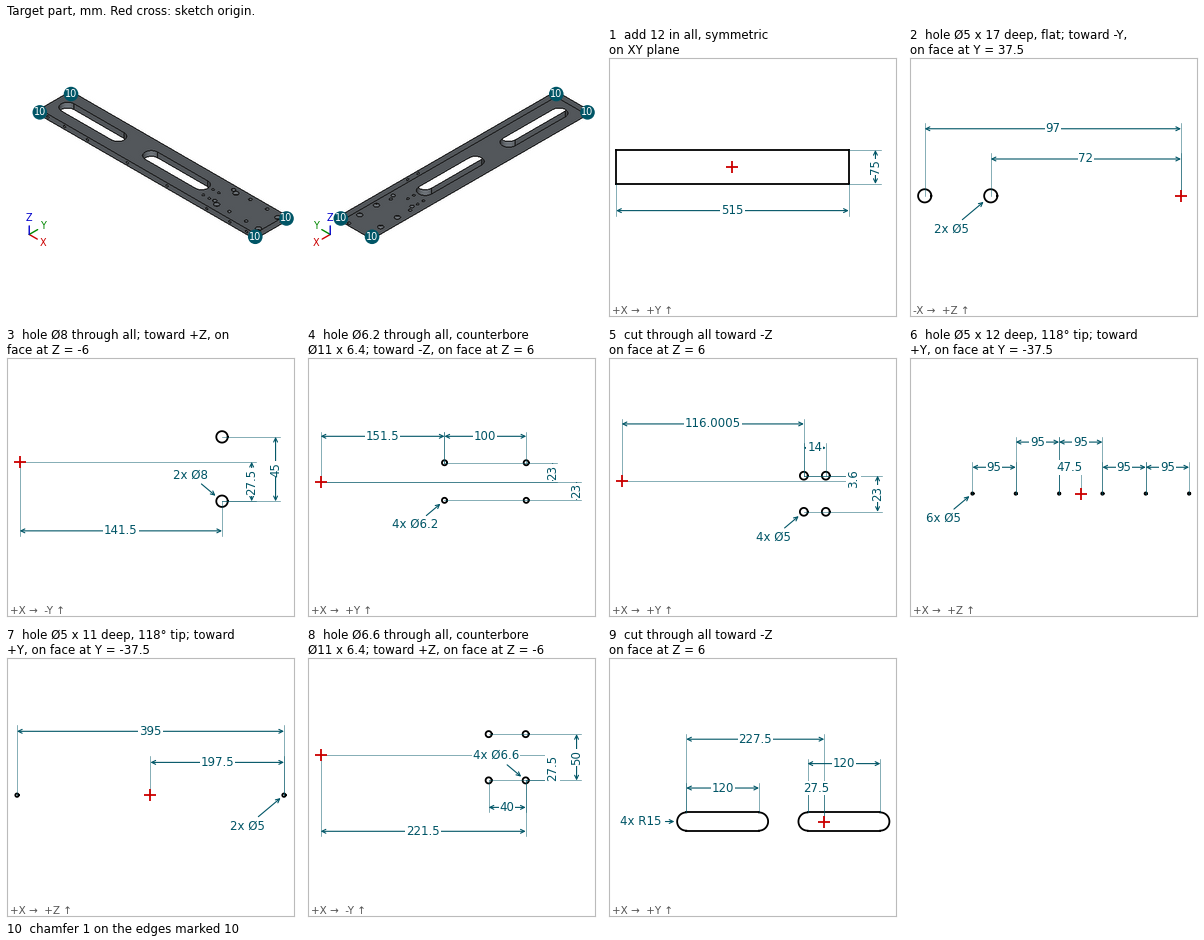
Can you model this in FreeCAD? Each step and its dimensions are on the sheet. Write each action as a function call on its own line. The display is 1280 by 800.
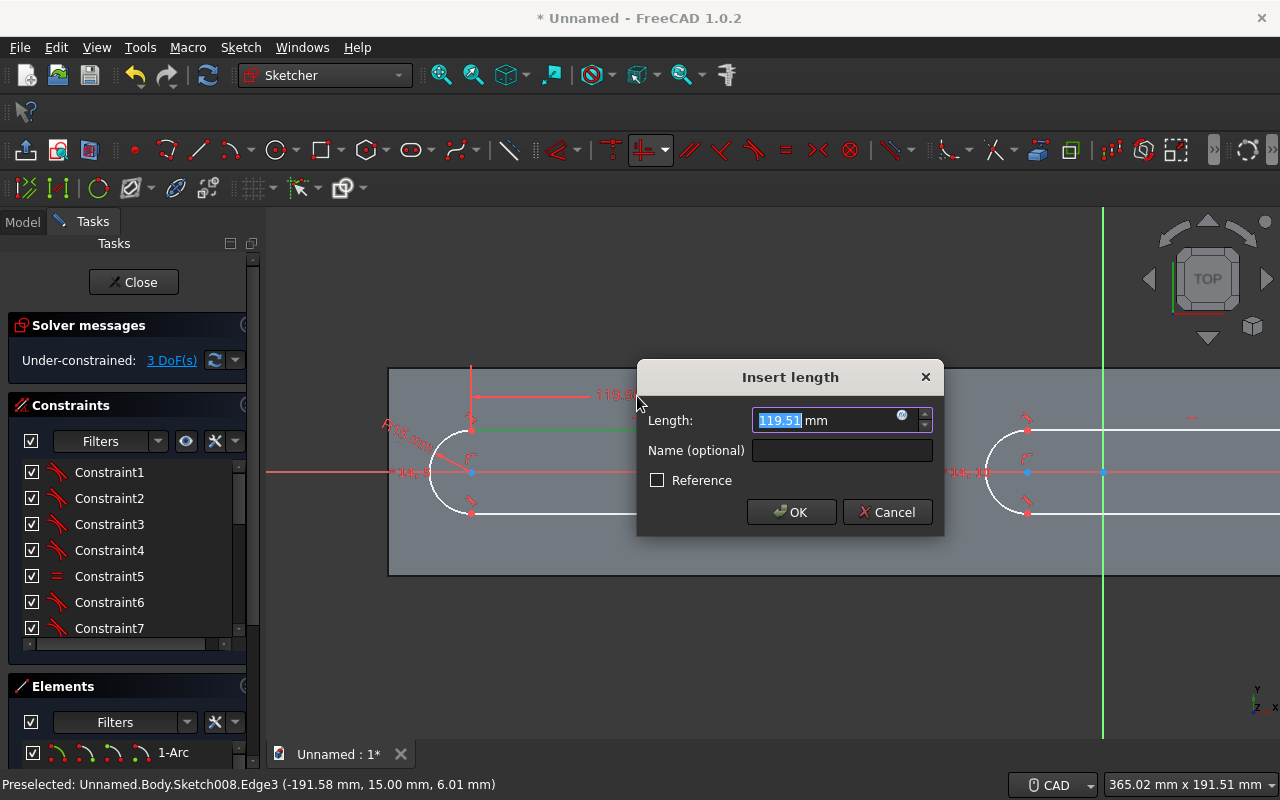
text(120)
key(Return)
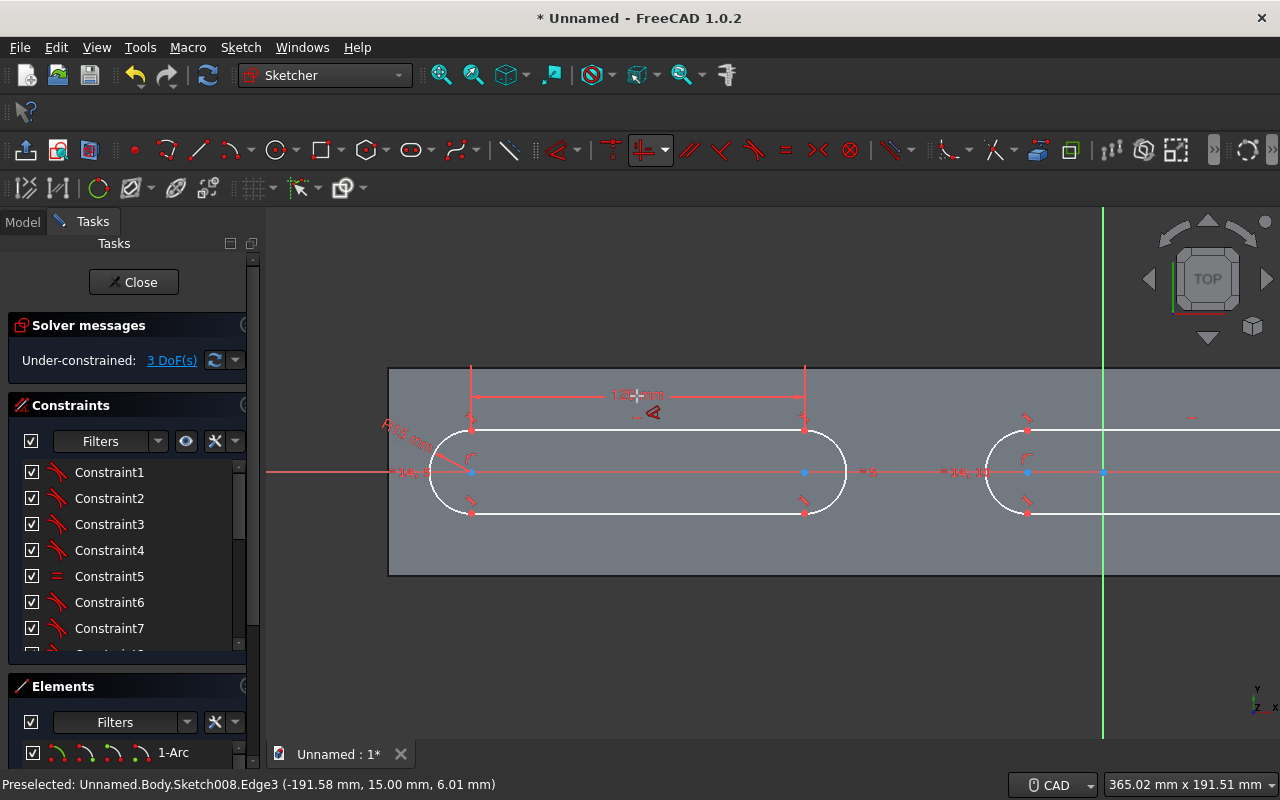
scroll(1094, 430, up, 2)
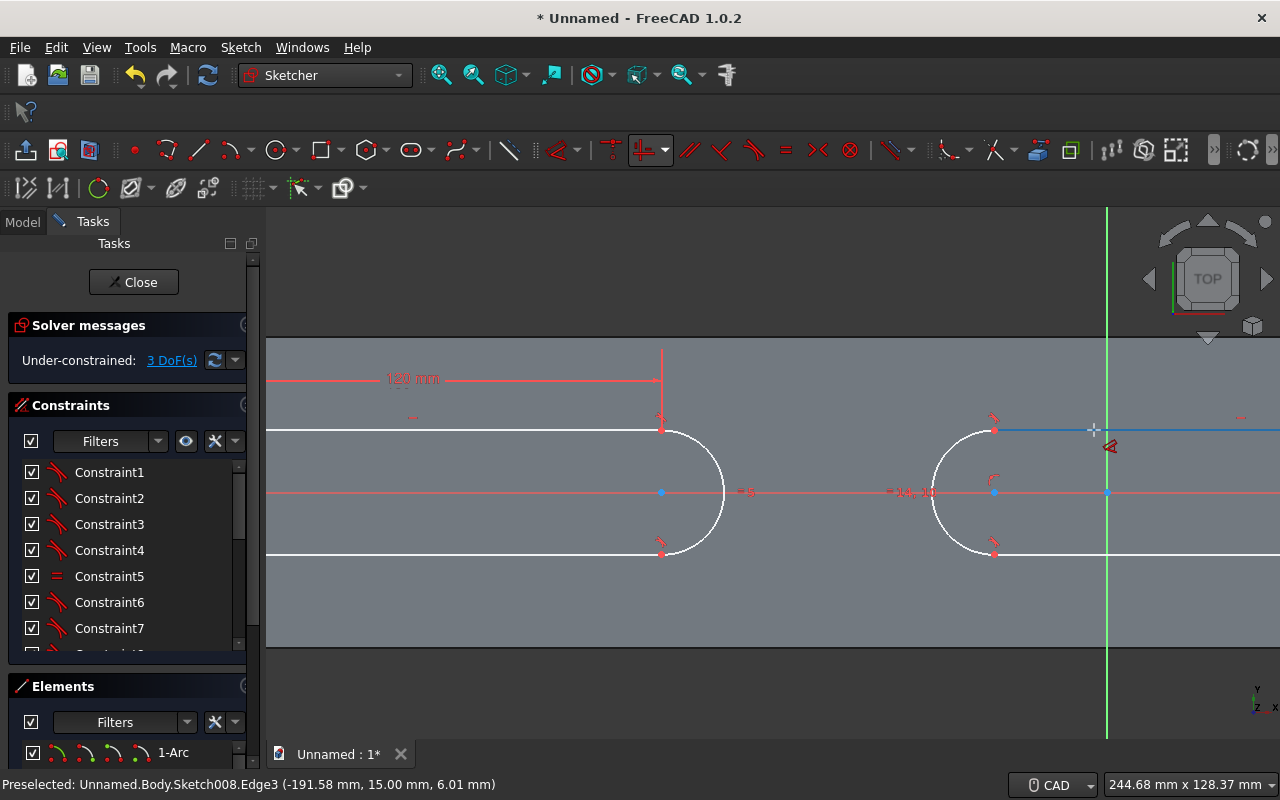
click(1093, 430)
click(1055, 396)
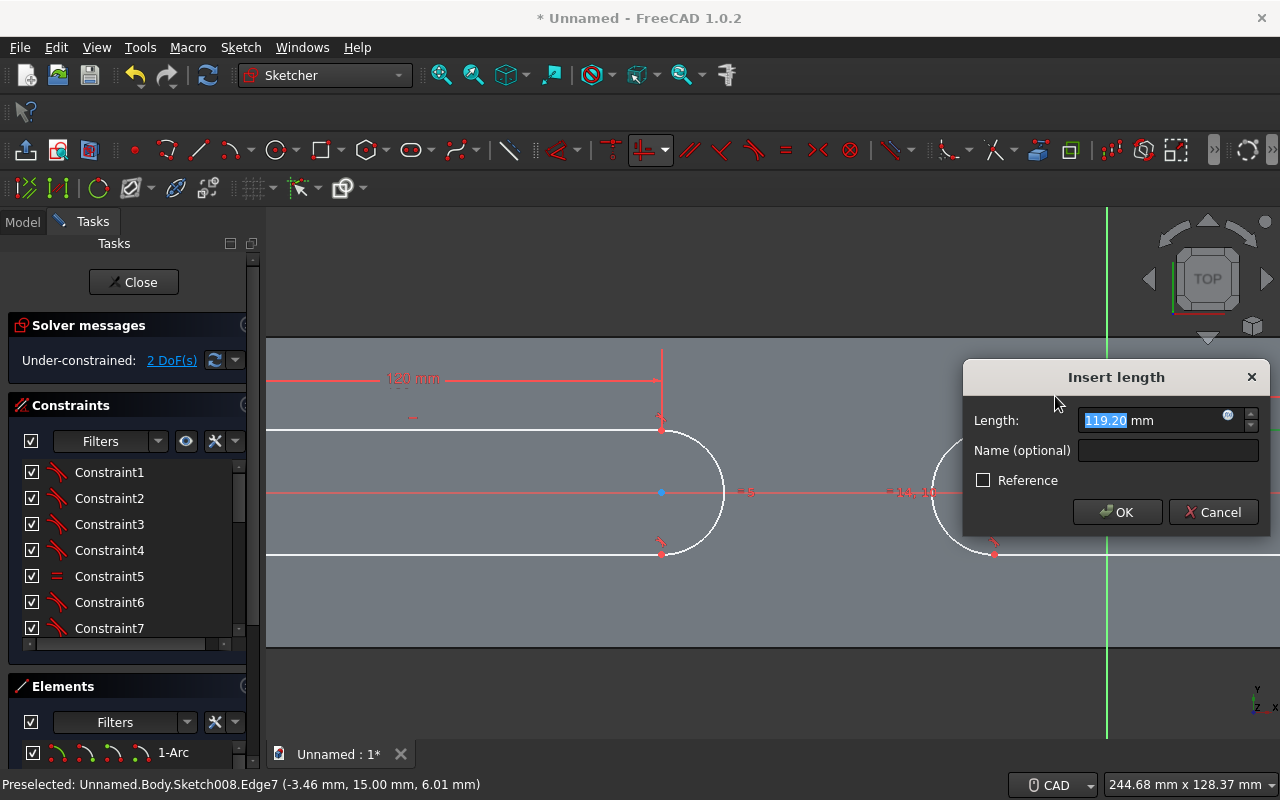
text(120)
key(Return)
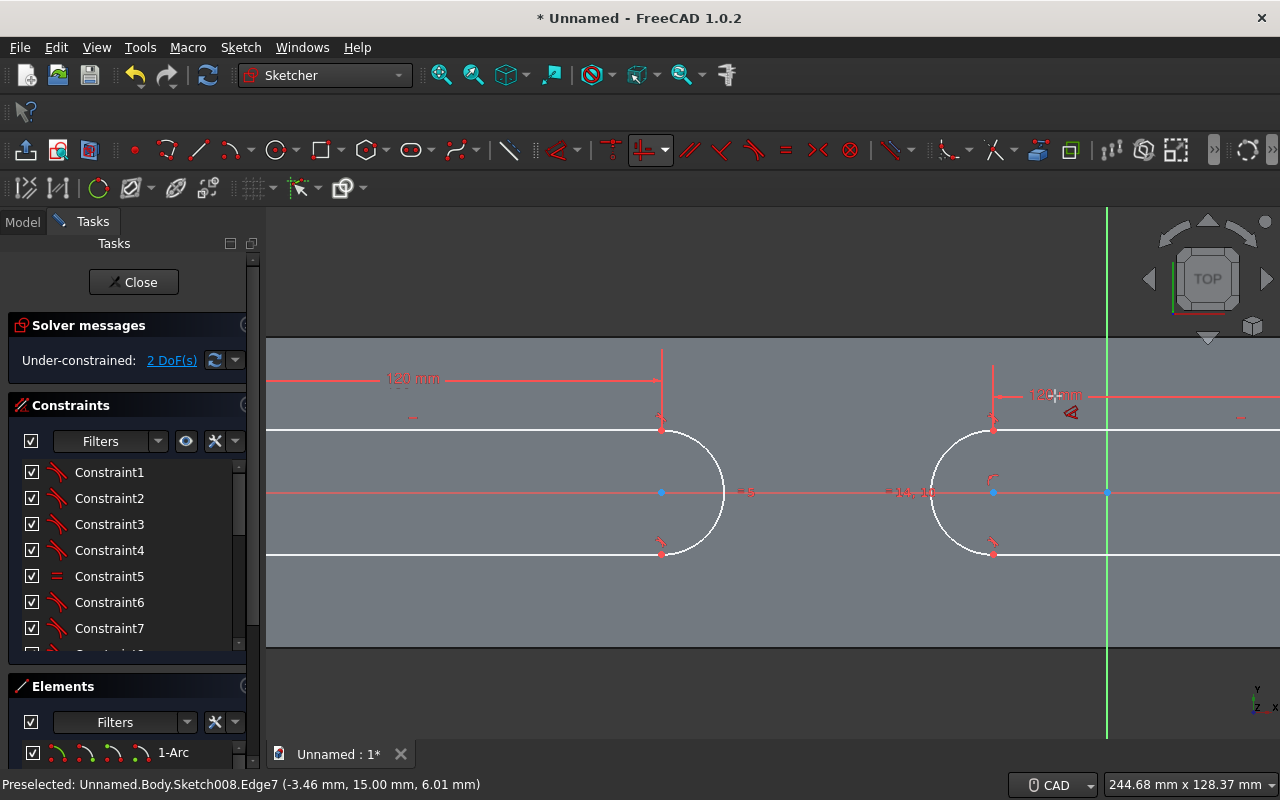
click(993, 430)
click(1050, 527)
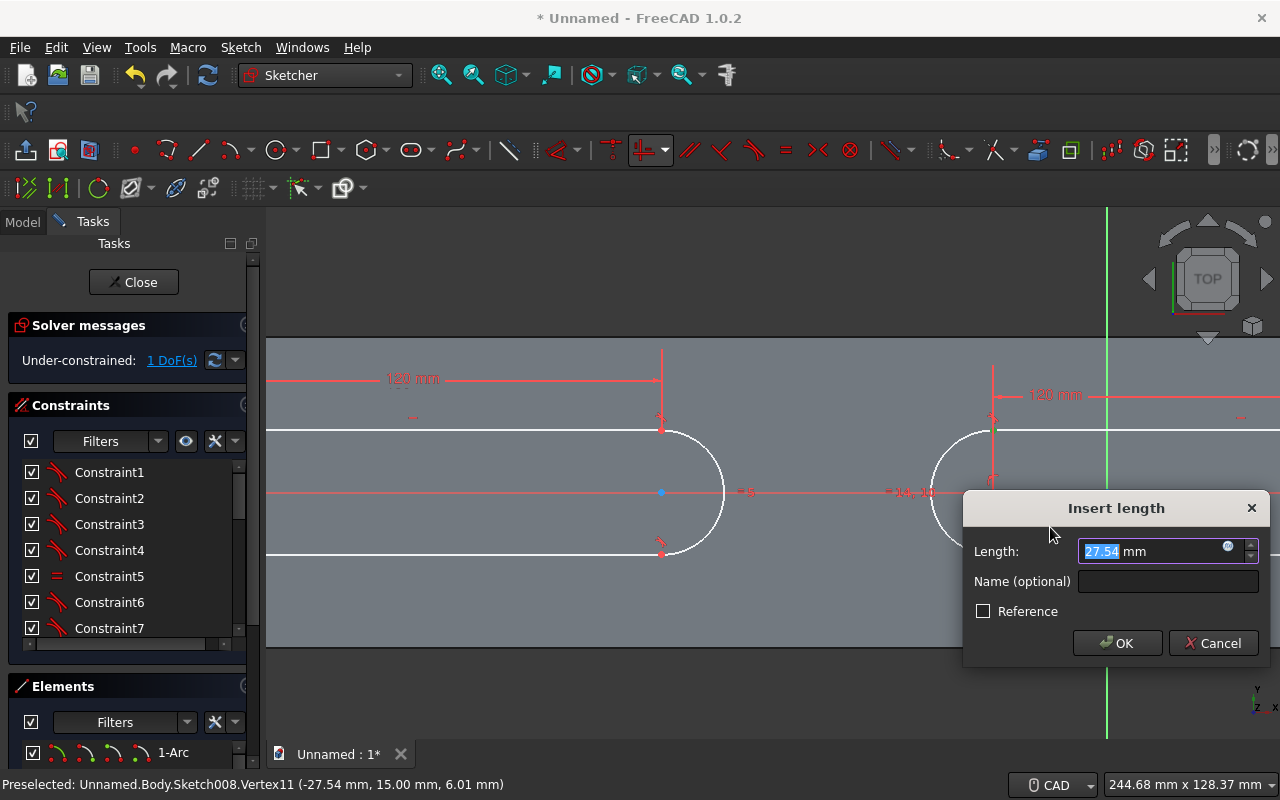
text(27.5)
key(Return)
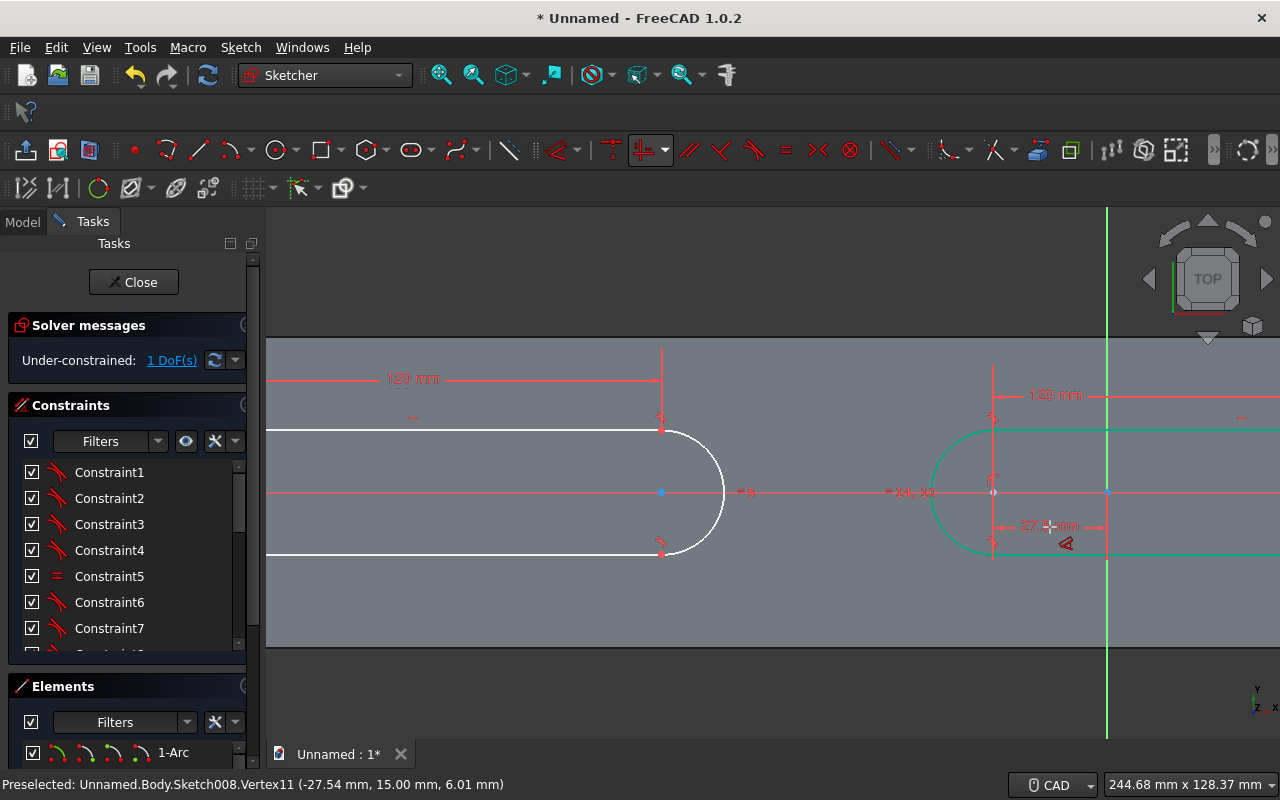
scroll(633, 462, down, 5)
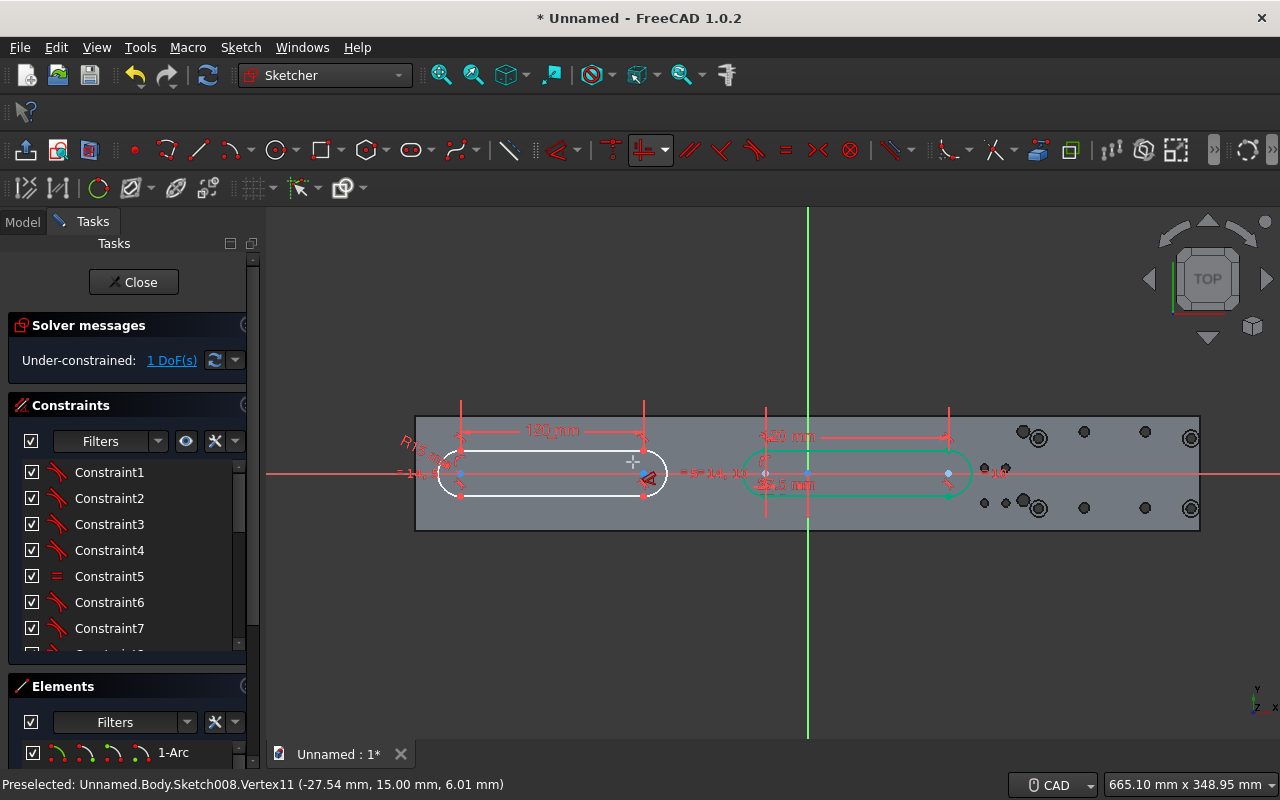
click(461, 451)
click(634, 417)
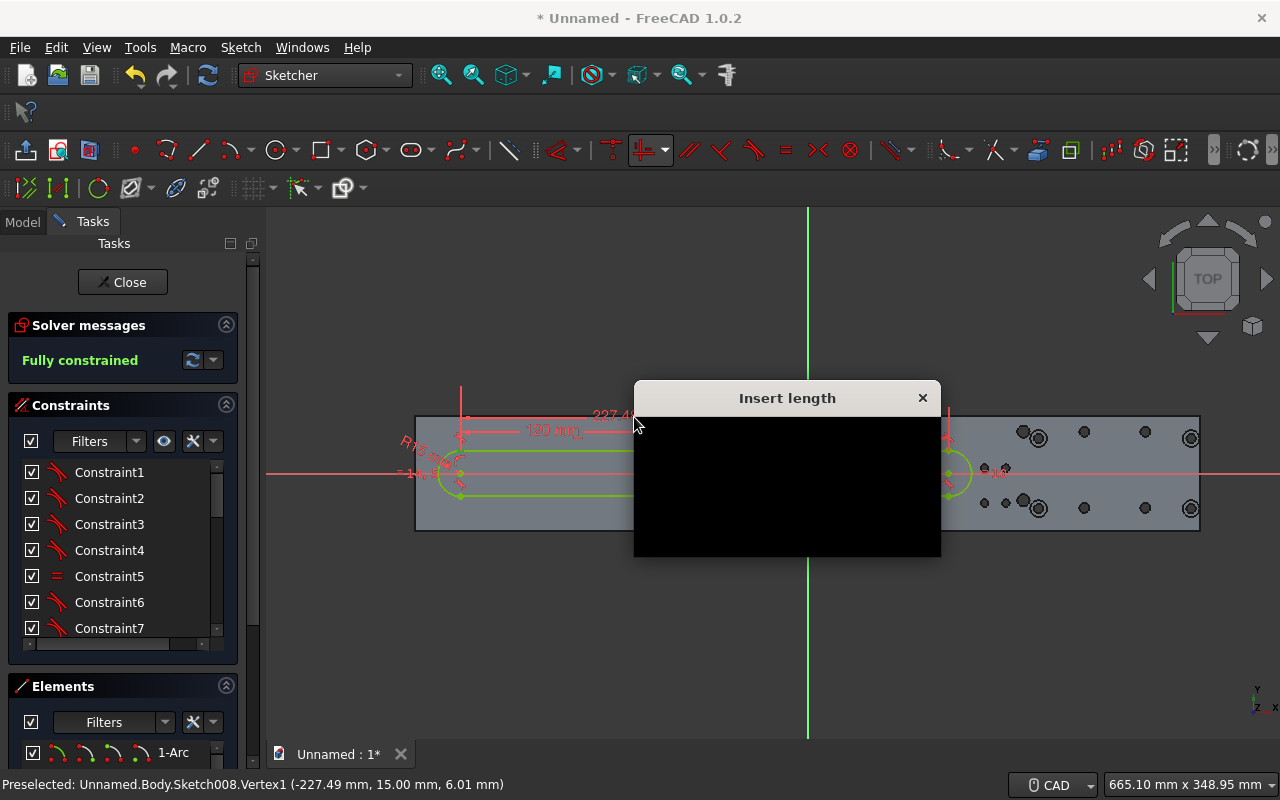
text(227.5)
key(Return)
key(Escape)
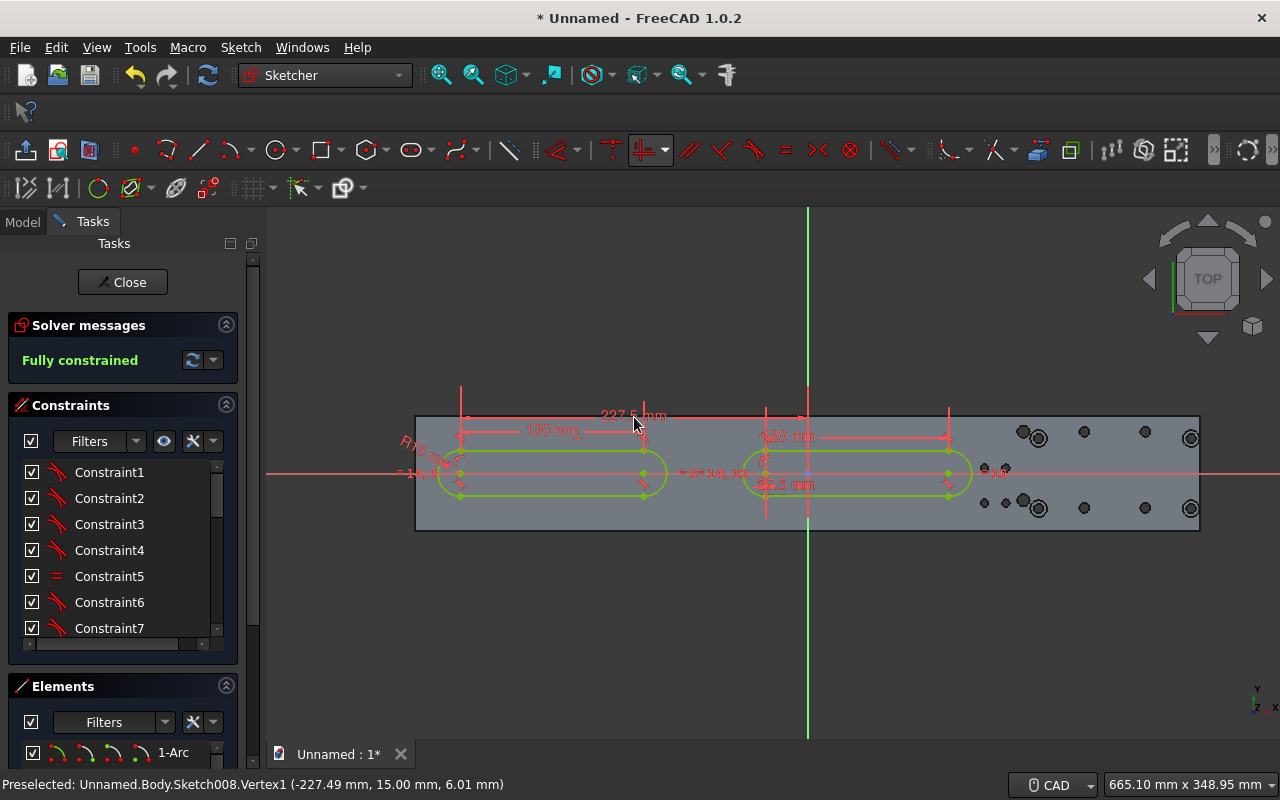
click(123, 282)